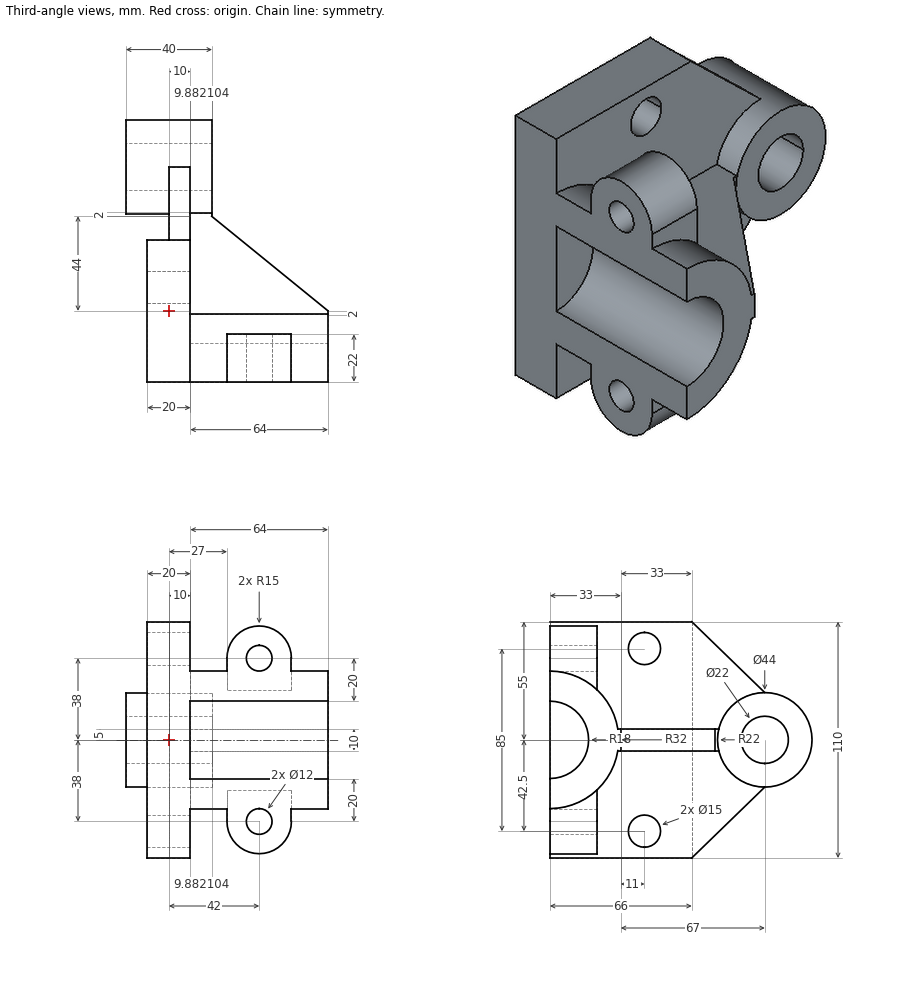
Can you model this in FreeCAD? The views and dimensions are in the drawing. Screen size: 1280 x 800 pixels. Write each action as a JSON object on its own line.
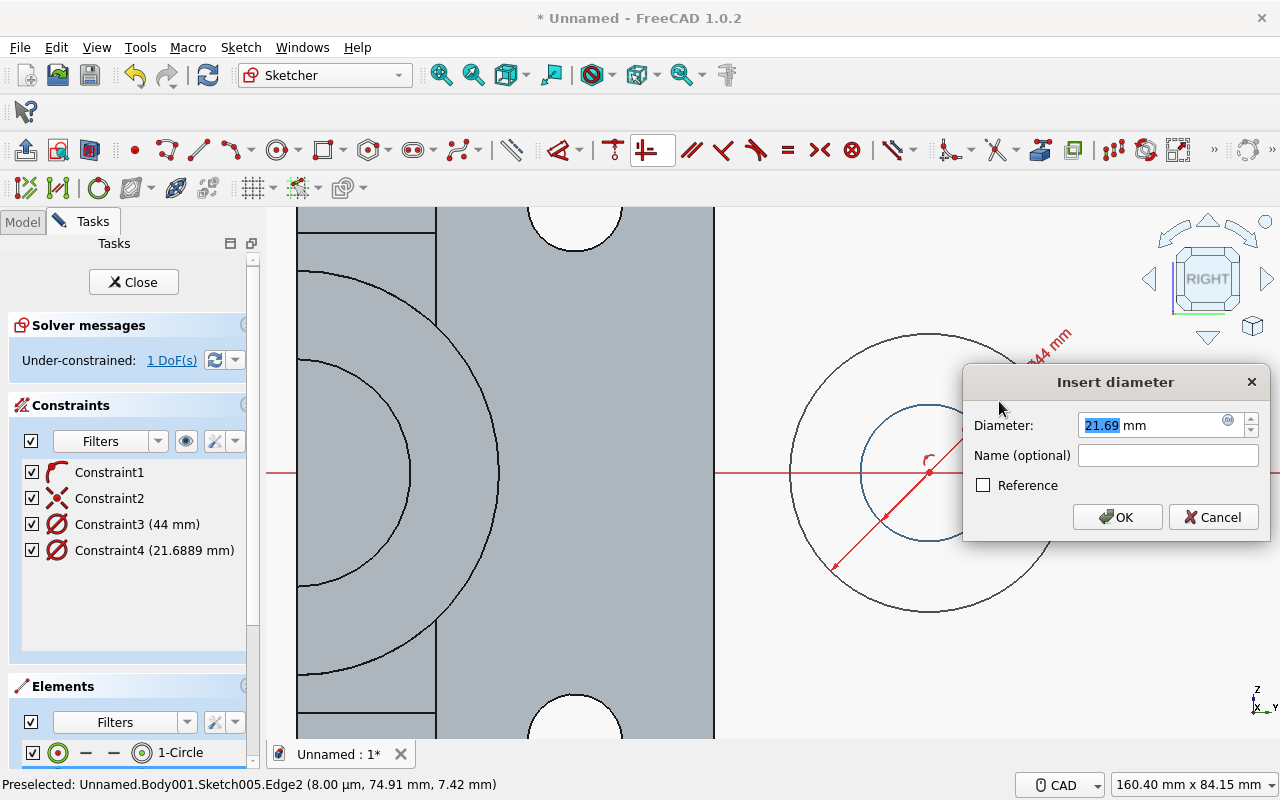
{"action": "type", "text": "22"}
{"action": "key", "text": "Return"}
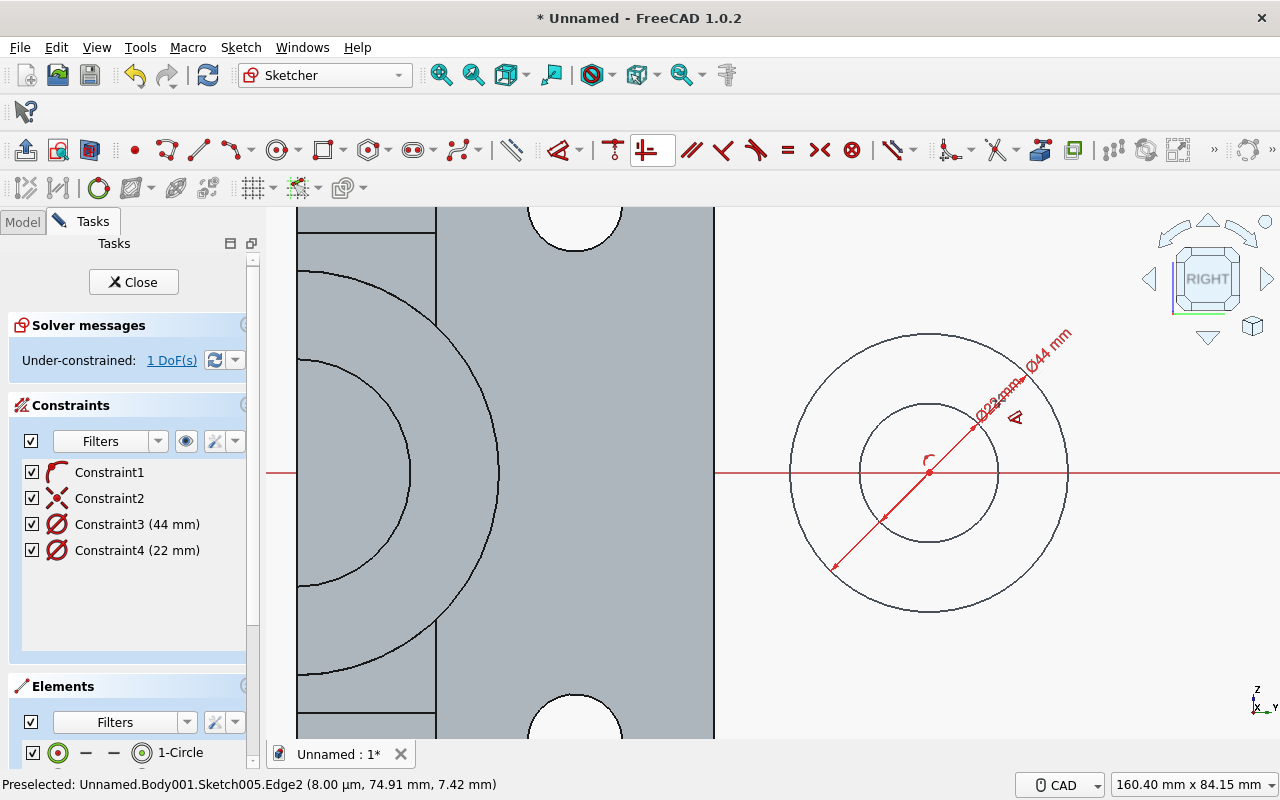
{"action": "left_click", "coordinate": [929, 473]}
{"action": "left_click", "coordinate": [717, 507]}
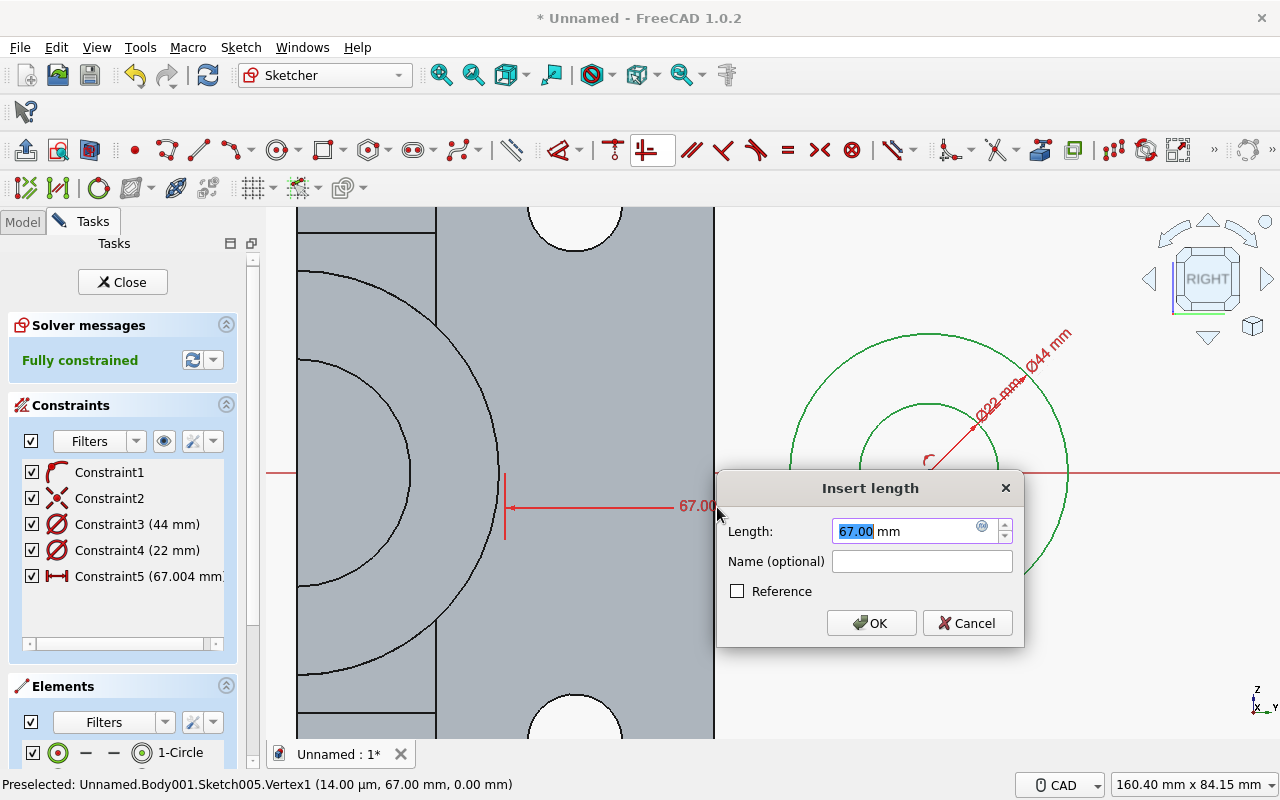
{"action": "type", "text": "67"}
{"action": "key", "text": "Return"}
{"action": "key", "text": "Escape"}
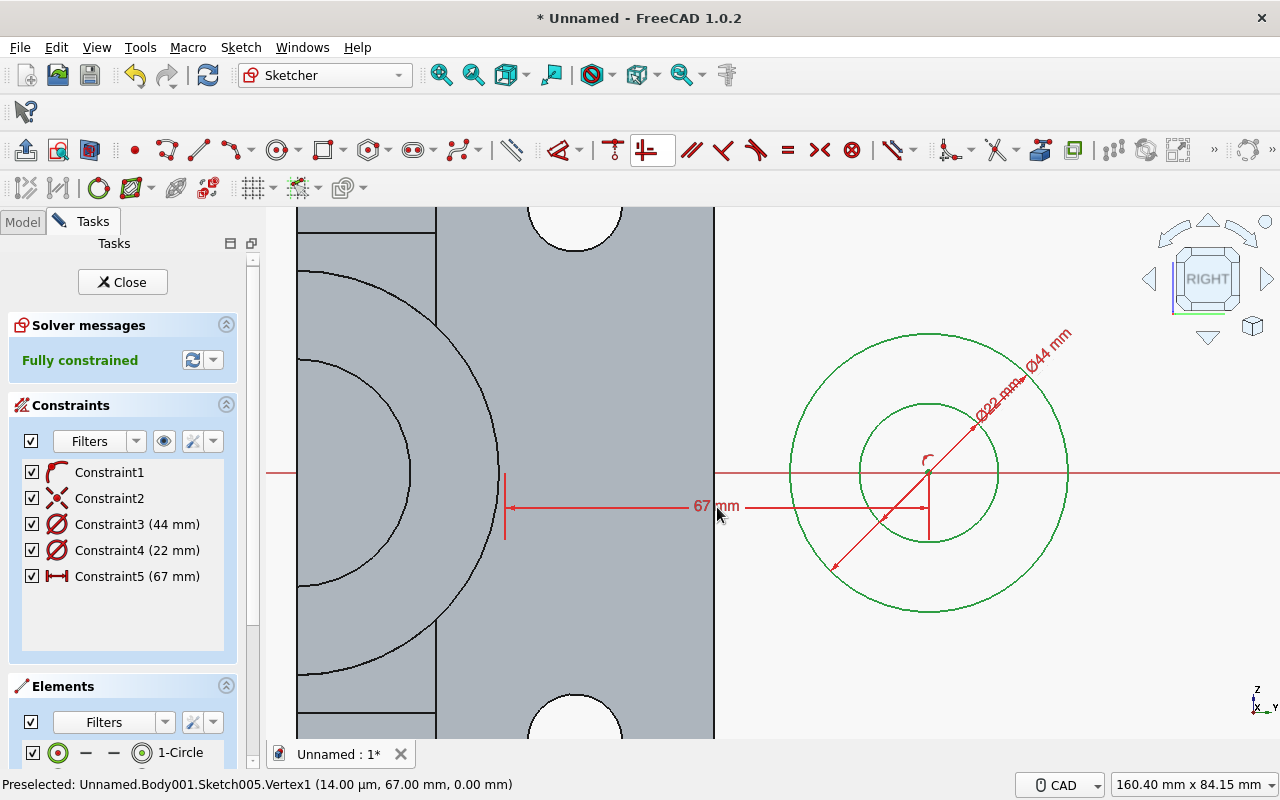
{"action": "left_click", "coordinate": [123, 282]}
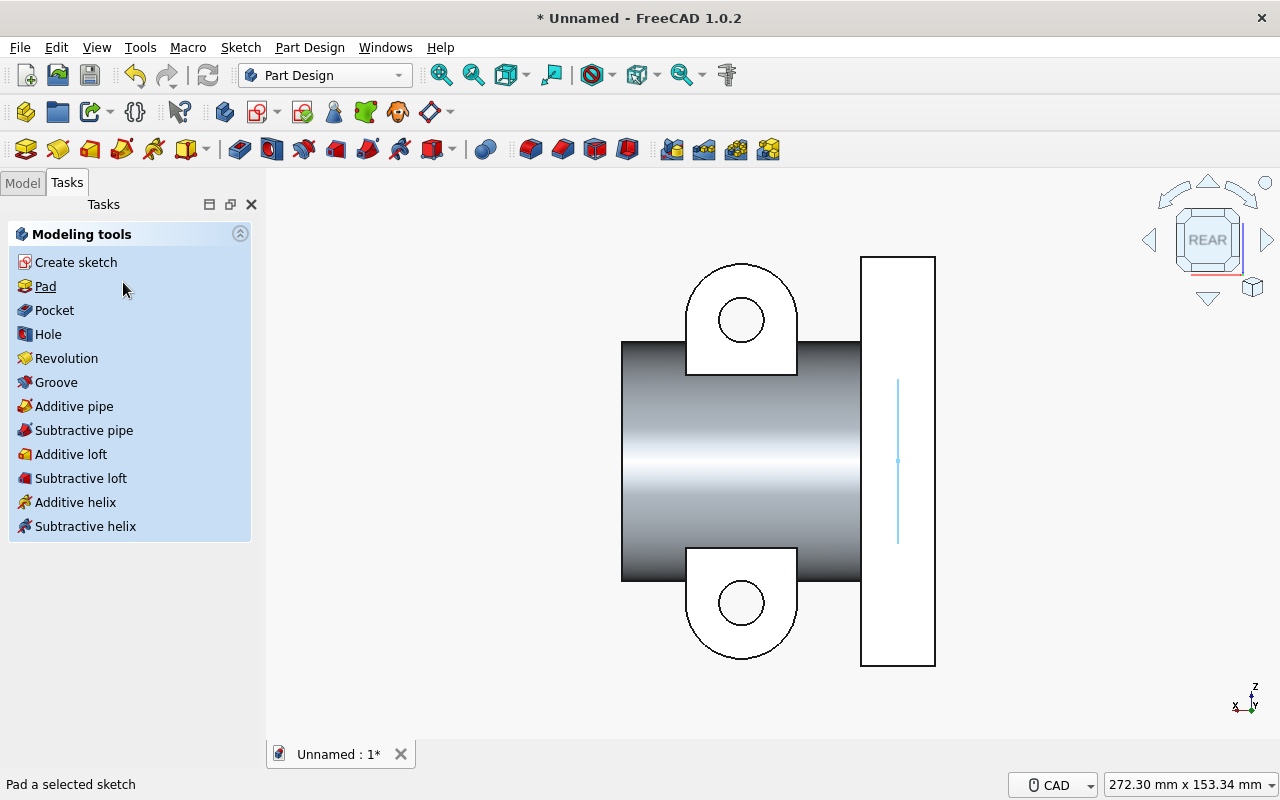
{"action": "left_click", "coordinate": [26, 150]}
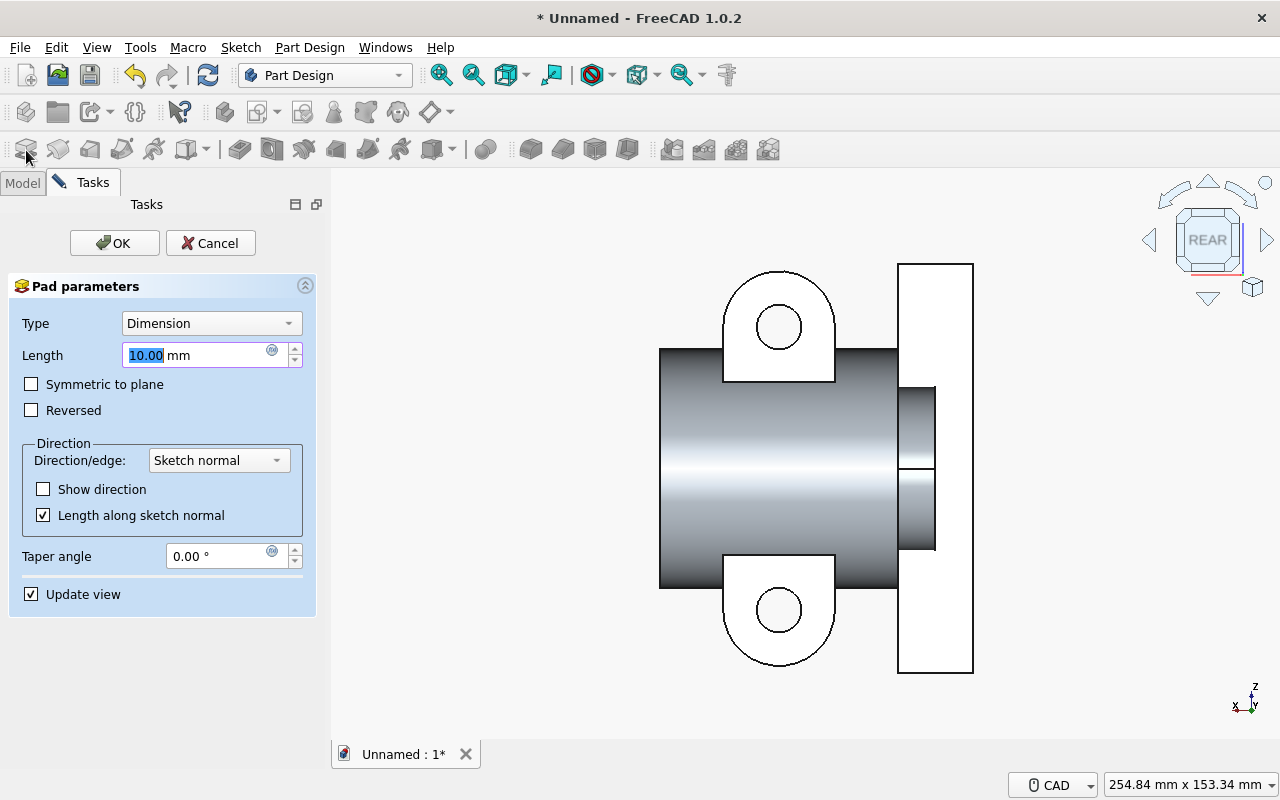
{"action": "type", "text": "40"}
{"action": "key", "text": "Tab"}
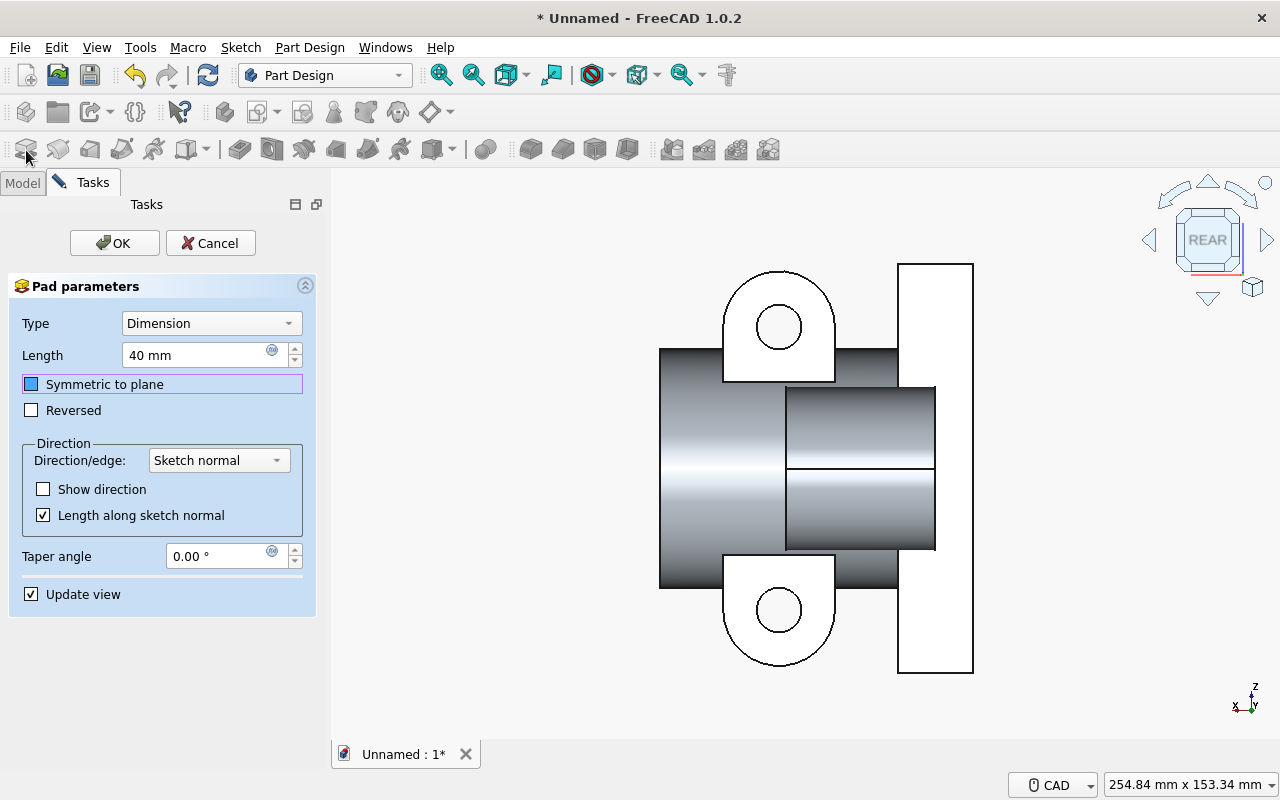
{"action": "left_click", "coordinate": [30, 384]}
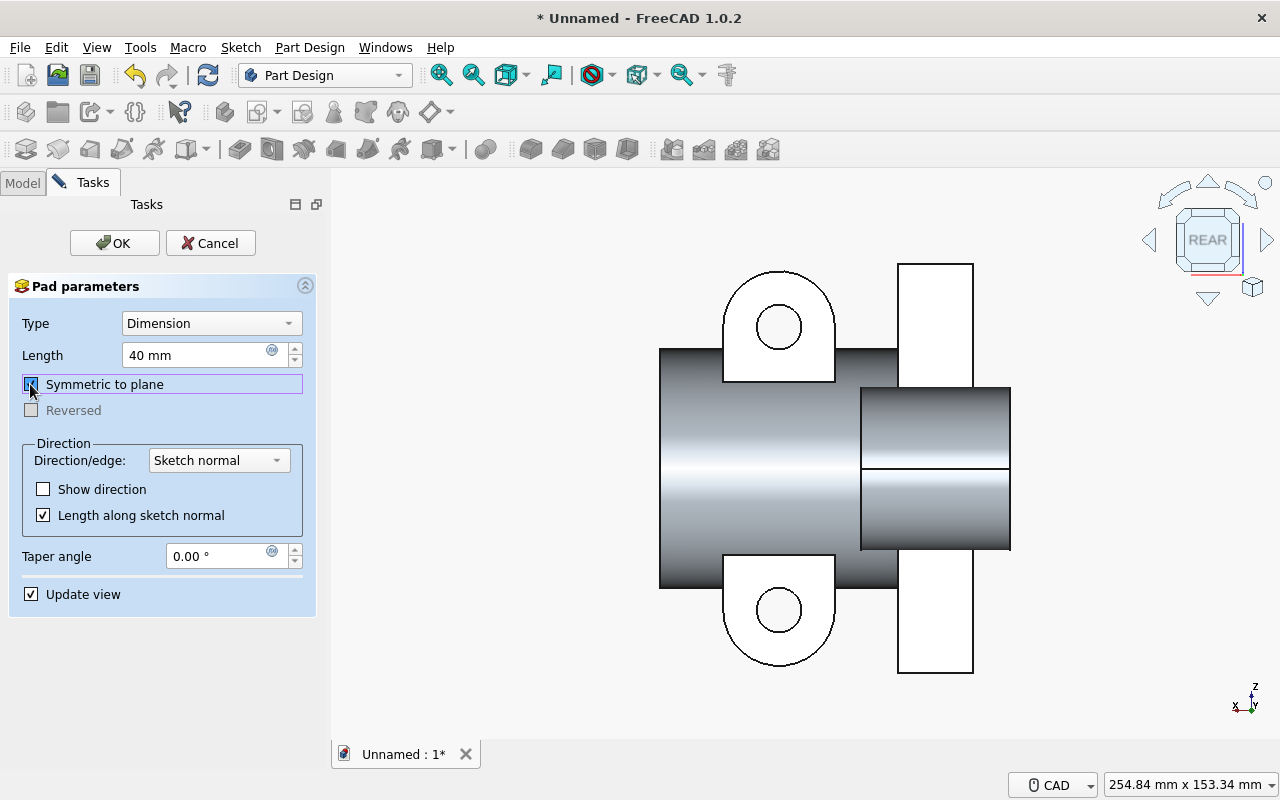
{"action": "left_click", "coordinate": [115, 243]}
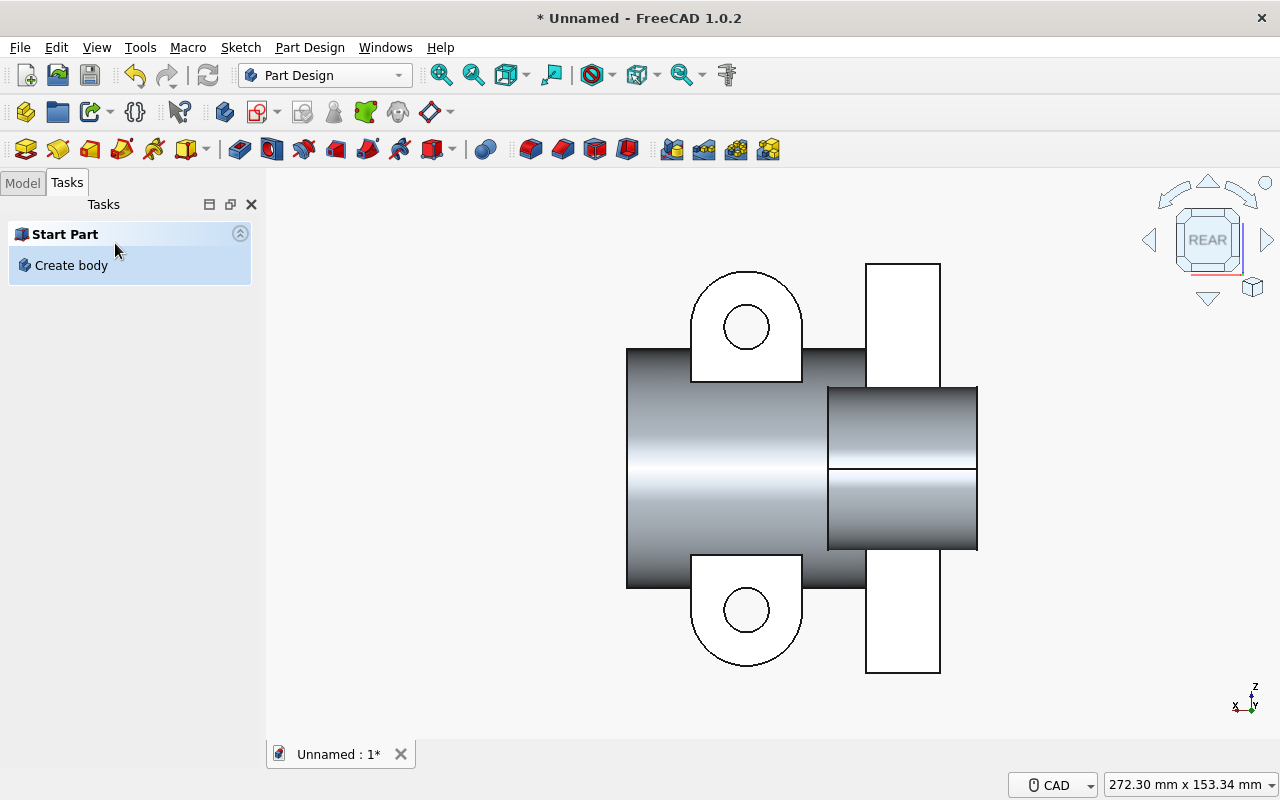
{"action": "key", "text": "v f"}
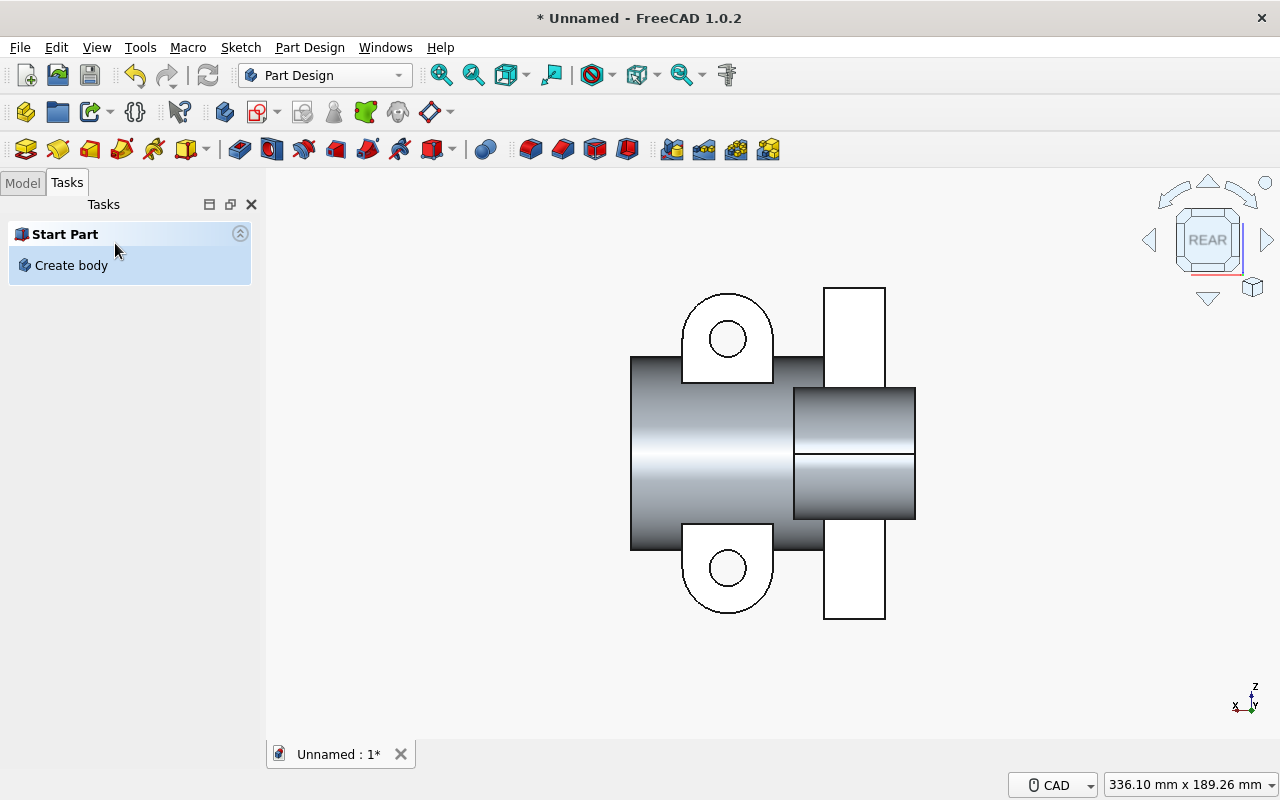
{"action": "left_click", "coordinate": [23, 182]}